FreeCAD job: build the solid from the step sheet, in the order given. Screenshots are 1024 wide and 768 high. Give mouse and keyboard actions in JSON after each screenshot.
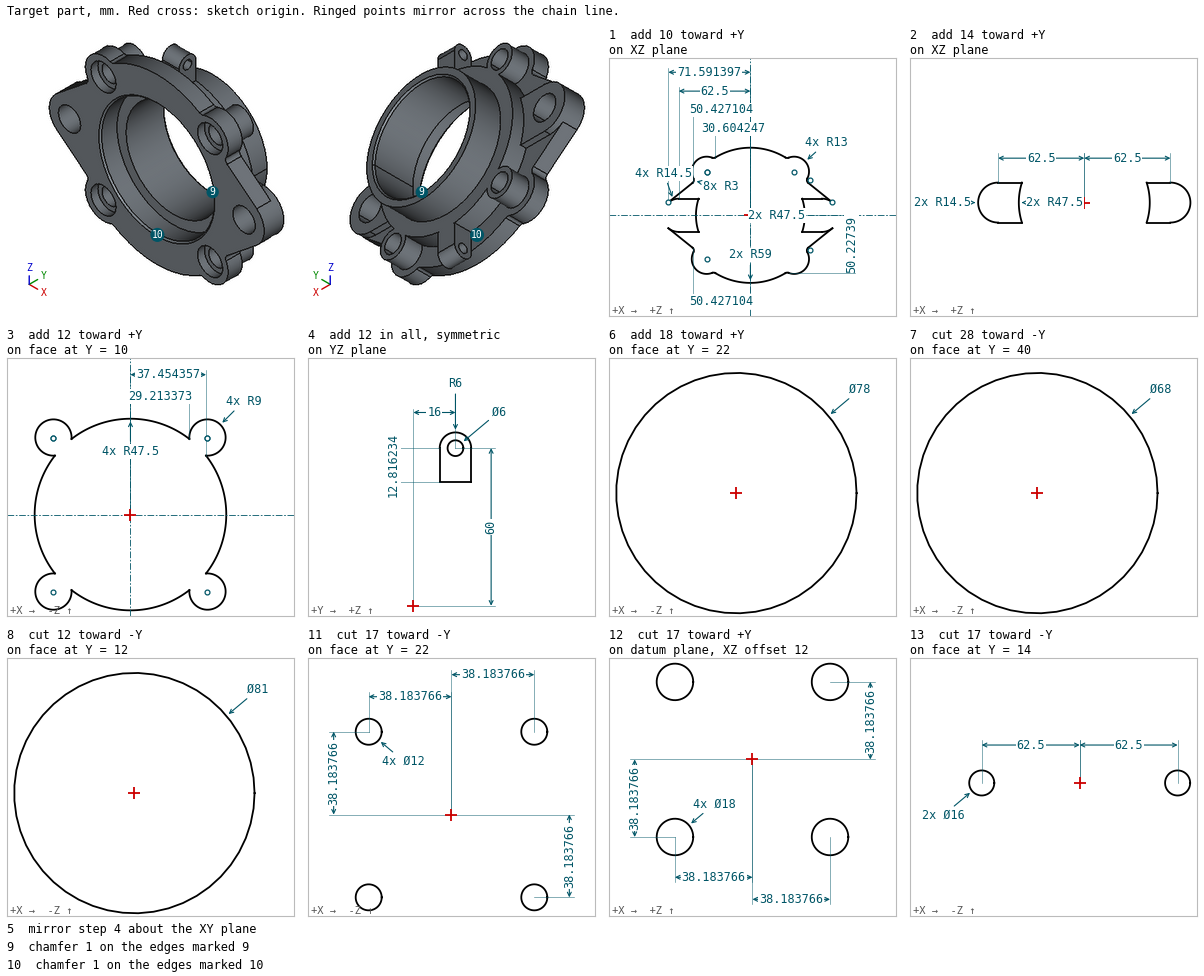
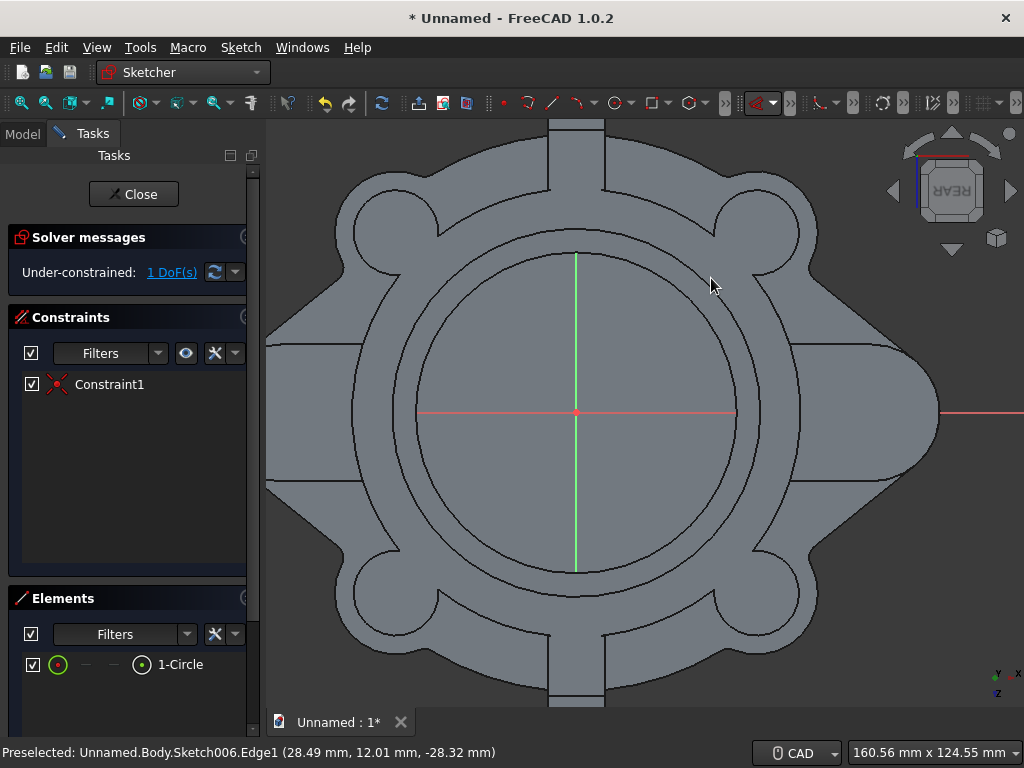
{"action": "key", "text": "d"}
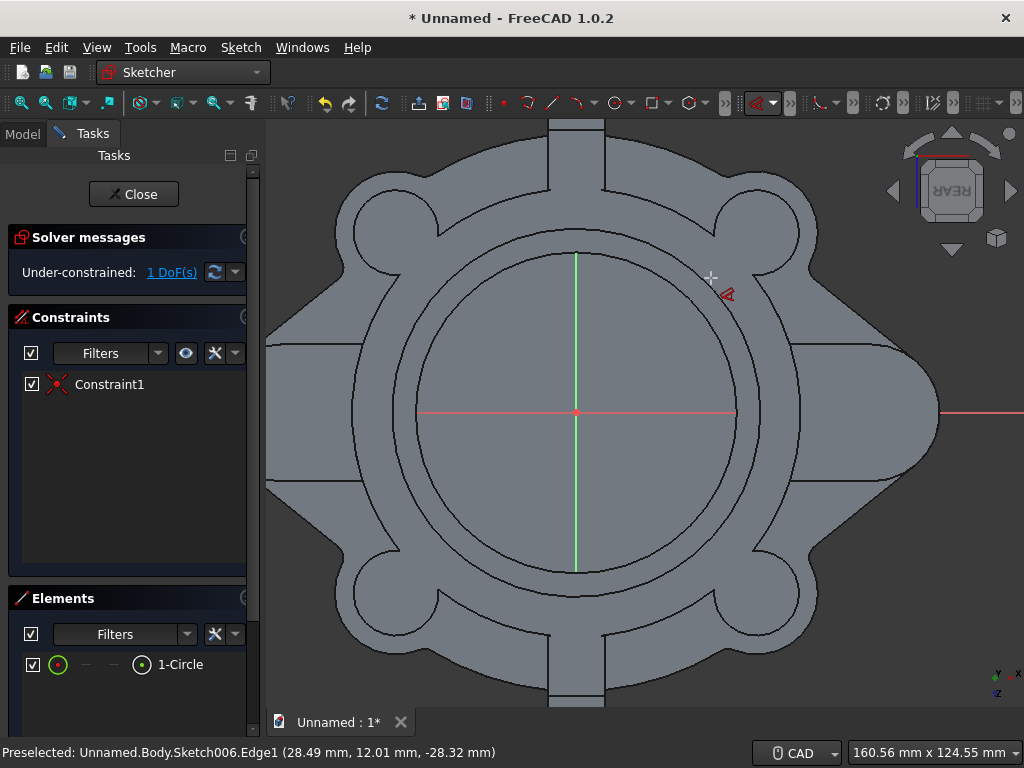
{"action": "left_click", "coordinate": [710, 278]}
{"action": "left_click", "coordinate": [733, 255]}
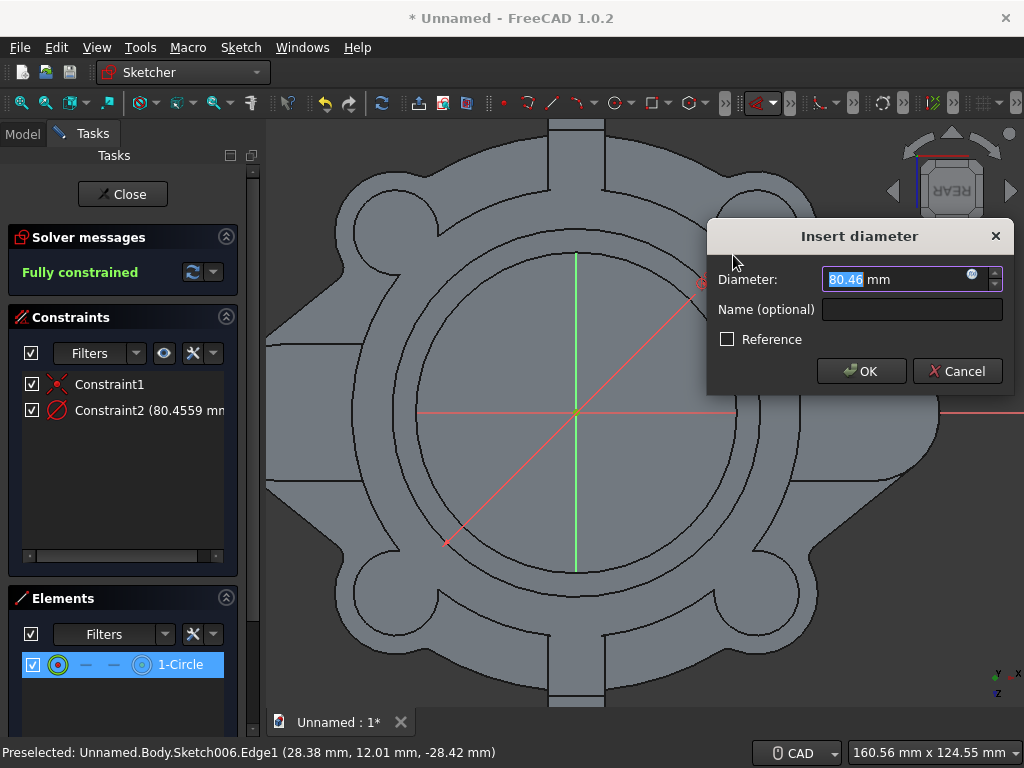
{"action": "type", "text": "81"}
{"action": "key", "text": "Return"}
{"action": "key", "text": "Escape"}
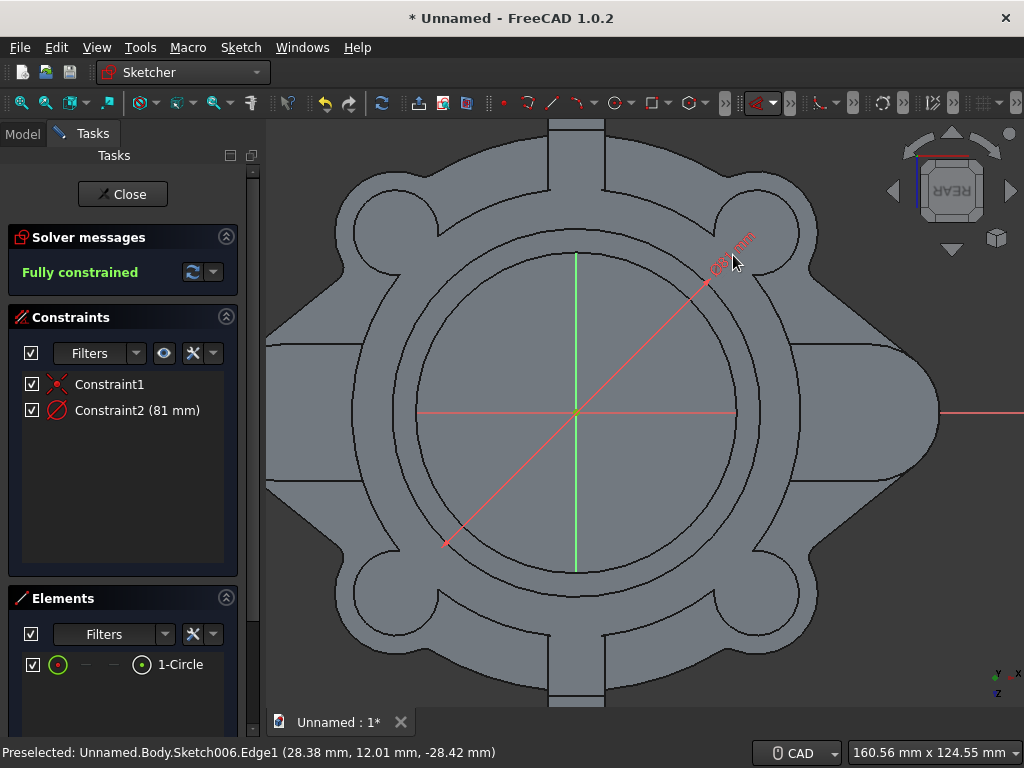
{"action": "left_click", "coordinate": [123, 194]}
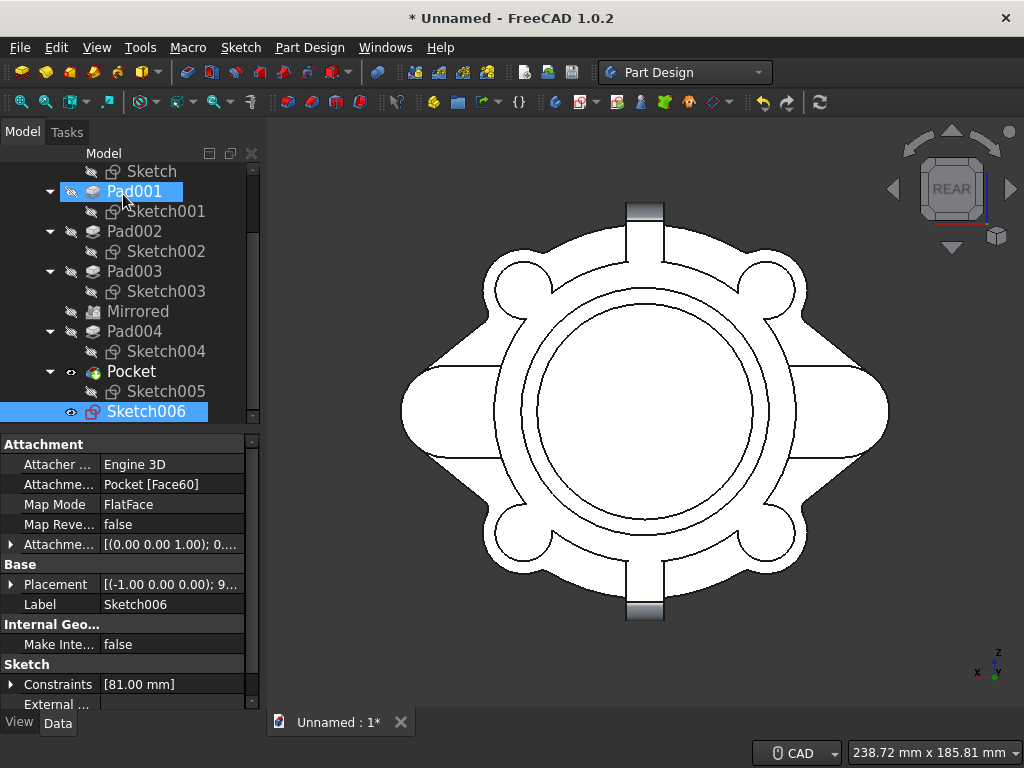
{"action": "left_click", "coordinate": [188, 72]}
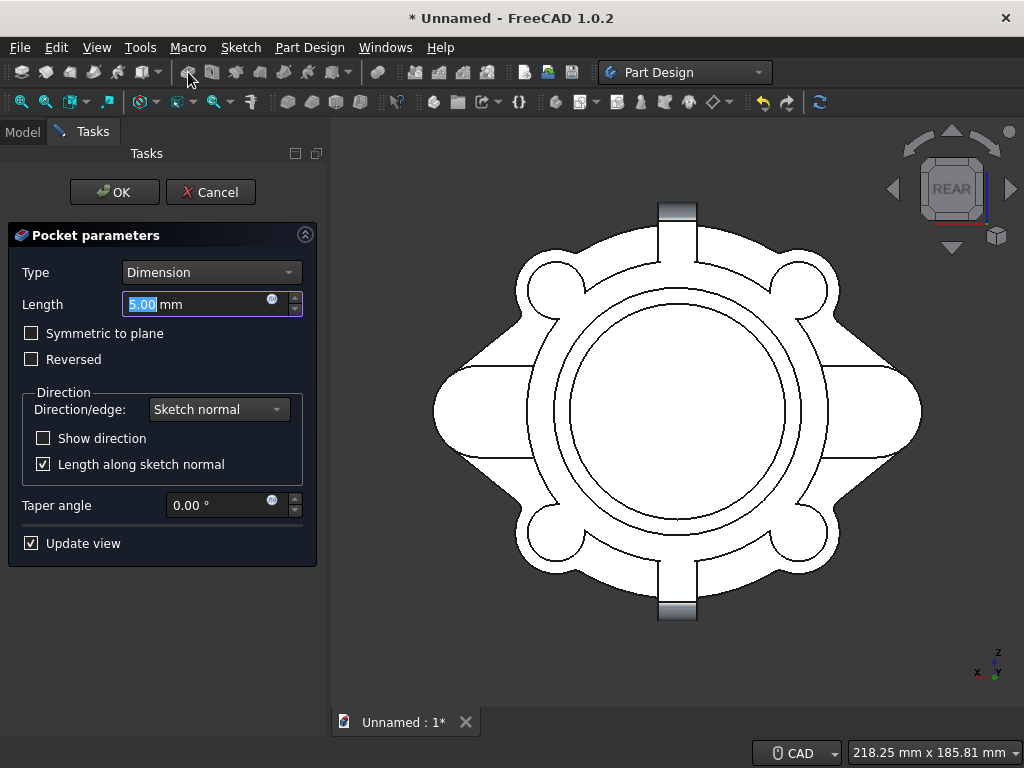
{"action": "type", "text": "12"}
{"action": "key", "text": "Tab"}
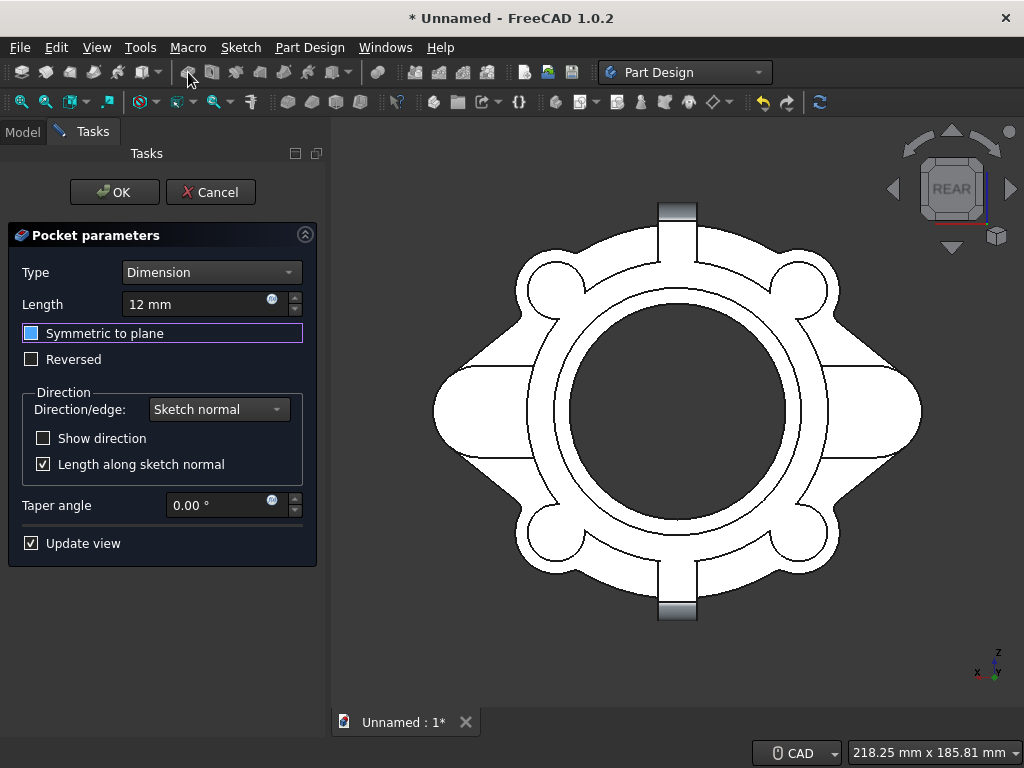
{"action": "left_click", "coordinate": [115, 192]}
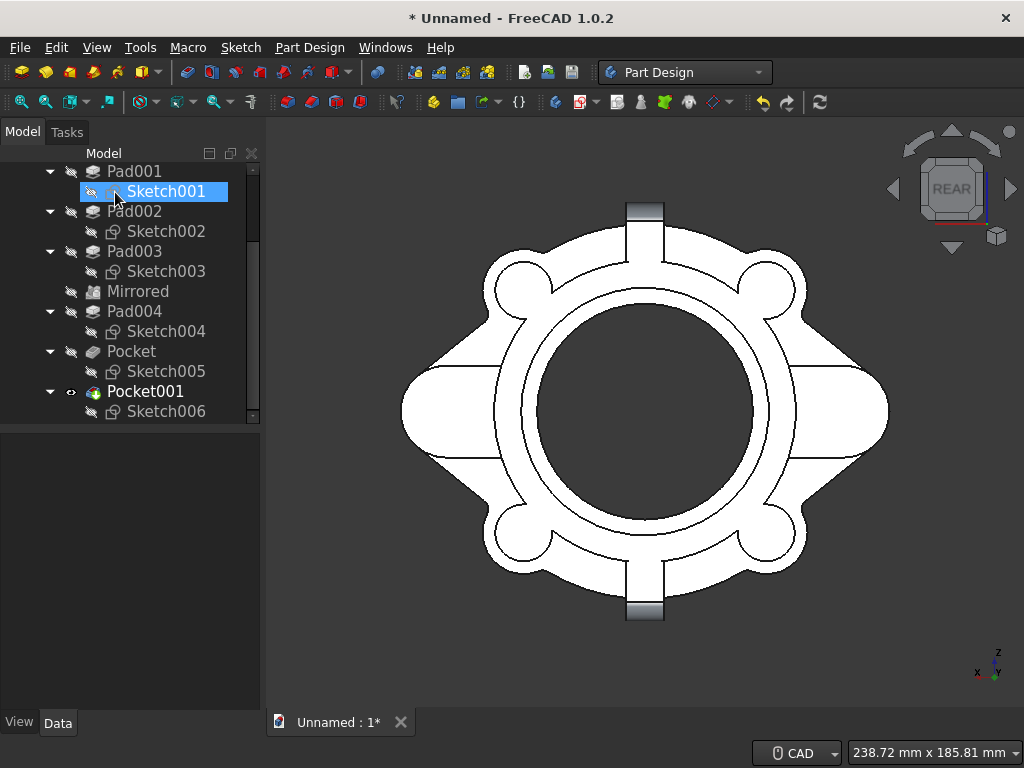
{"action": "left_click", "coordinate": [732, 347]}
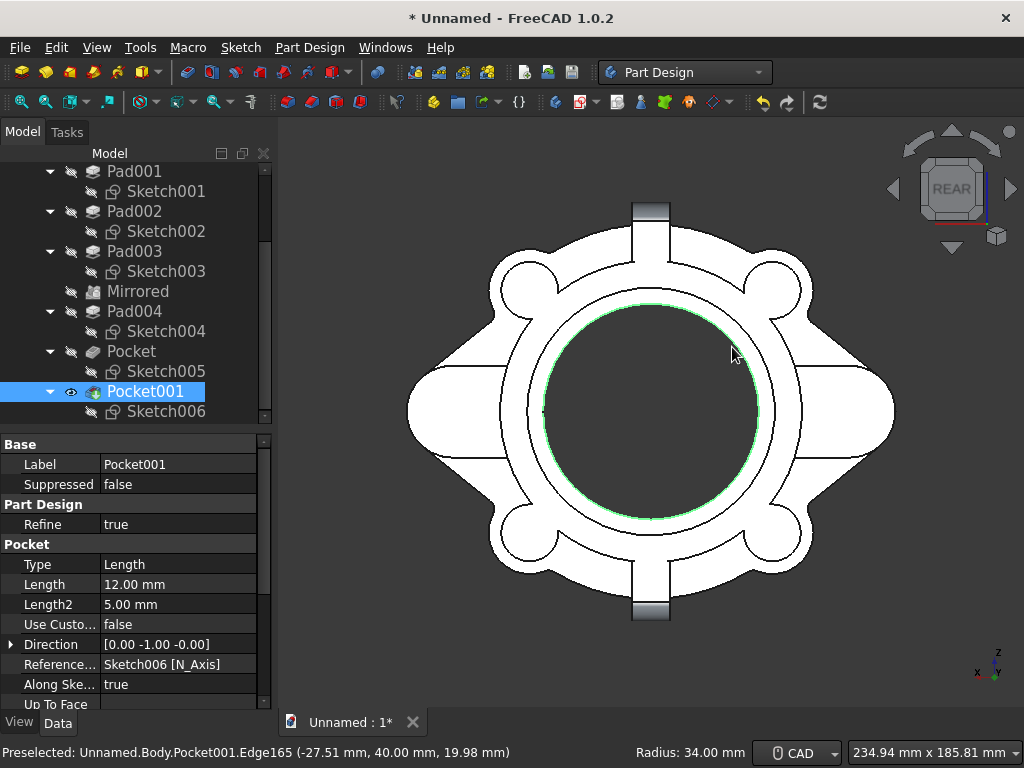
{"action": "left_click", "coordinate": [312, 102]}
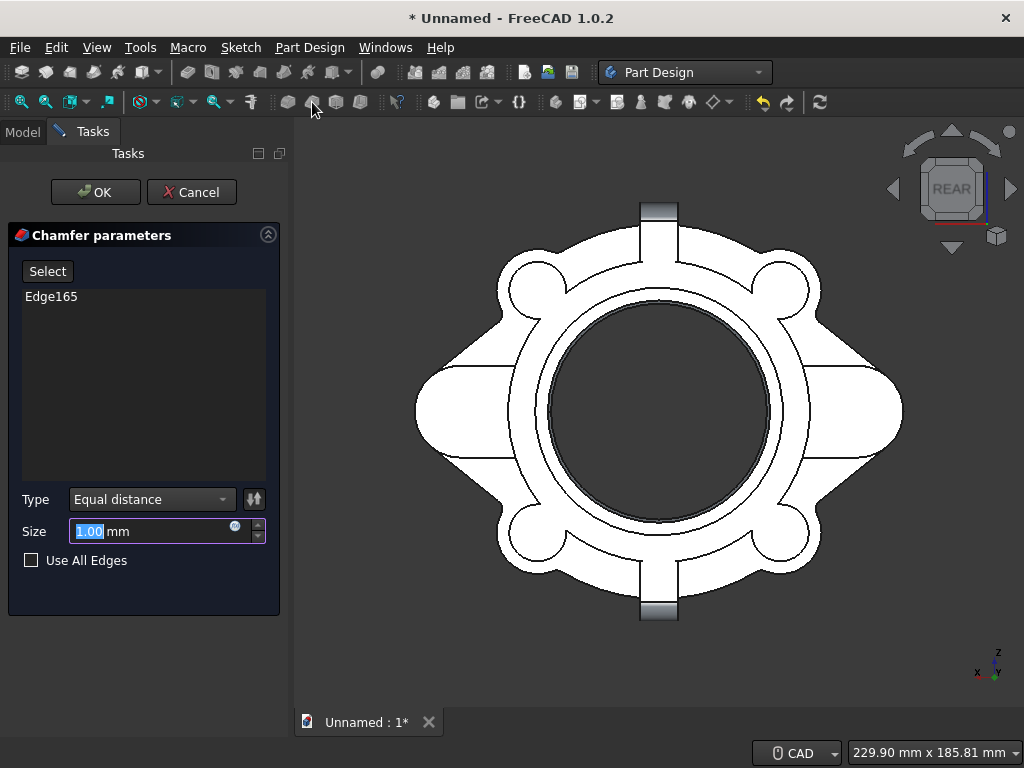
{"action": "type", "text": "1"}
{"action": "key", "text": "Tab"}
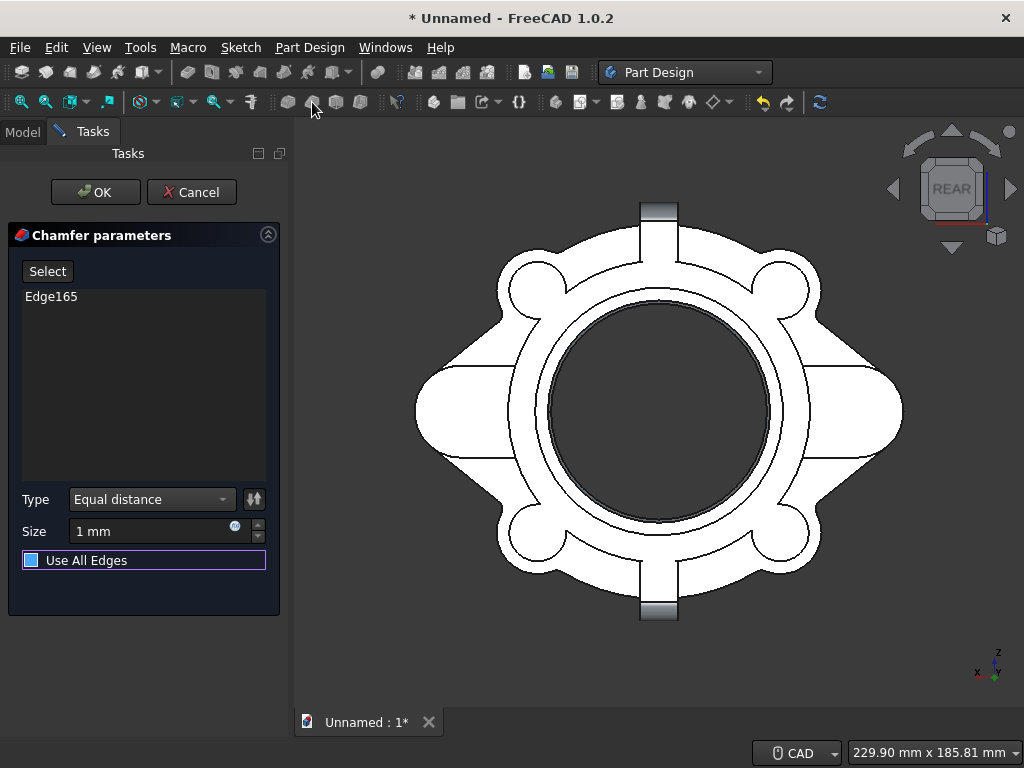
{"action": "left_click", "coordinate": [96, 192]}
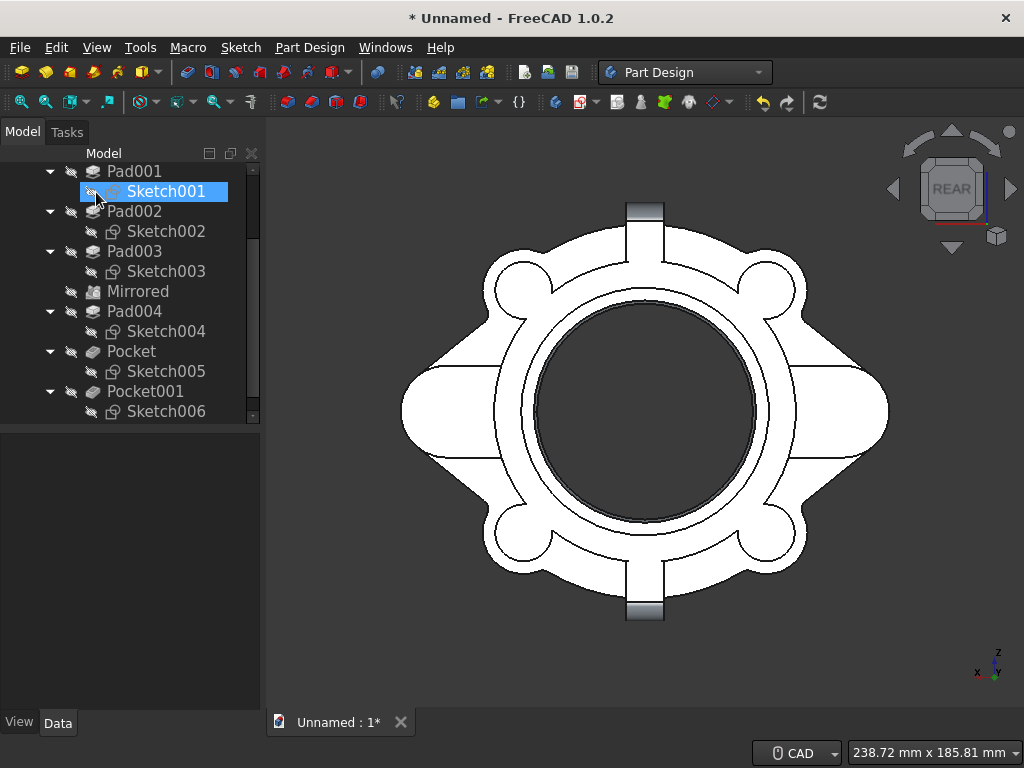
{"action": "key", "text": "0"}